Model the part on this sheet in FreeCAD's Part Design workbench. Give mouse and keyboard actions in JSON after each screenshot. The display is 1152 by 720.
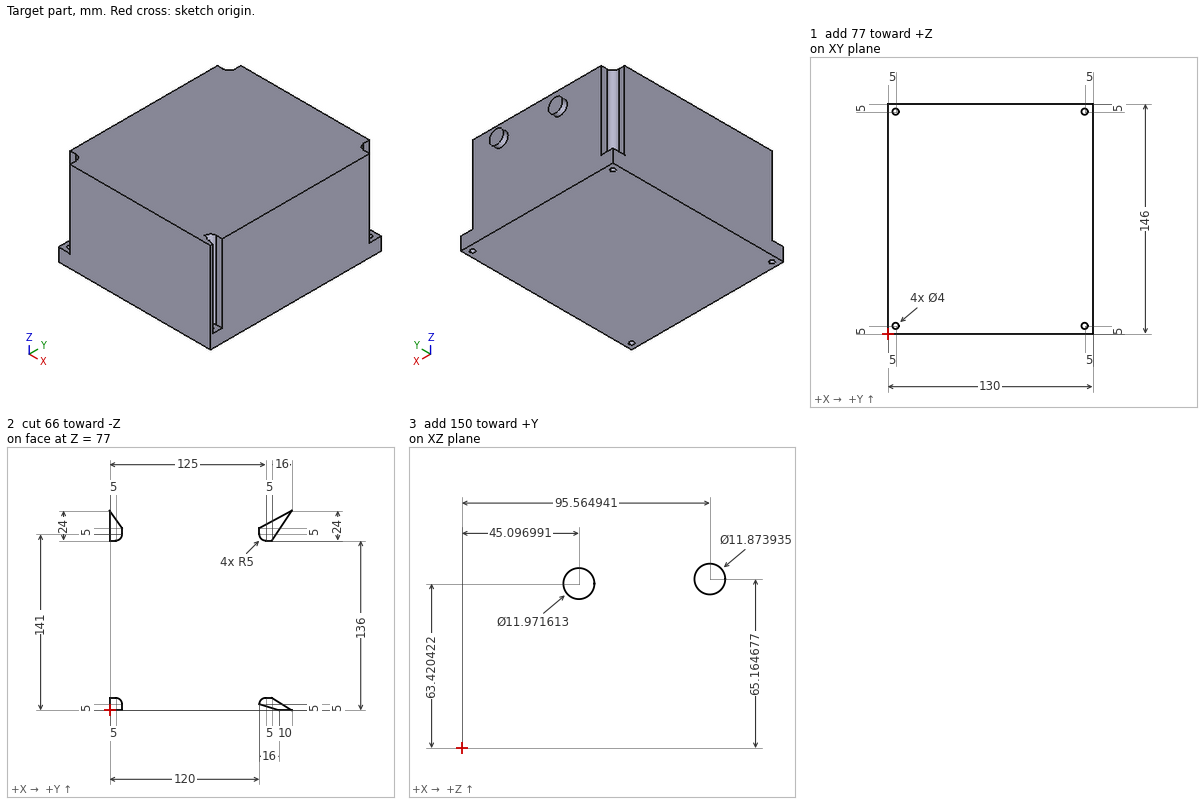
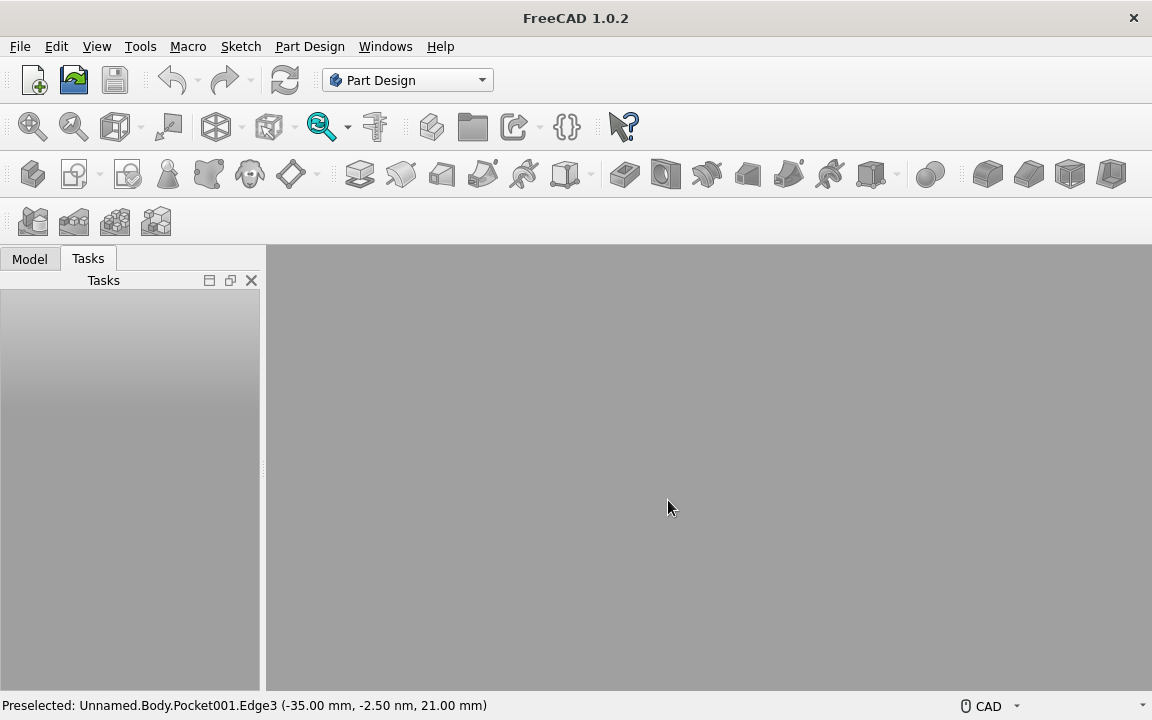
{"action": "left_click", "coordinate": [33, 80]}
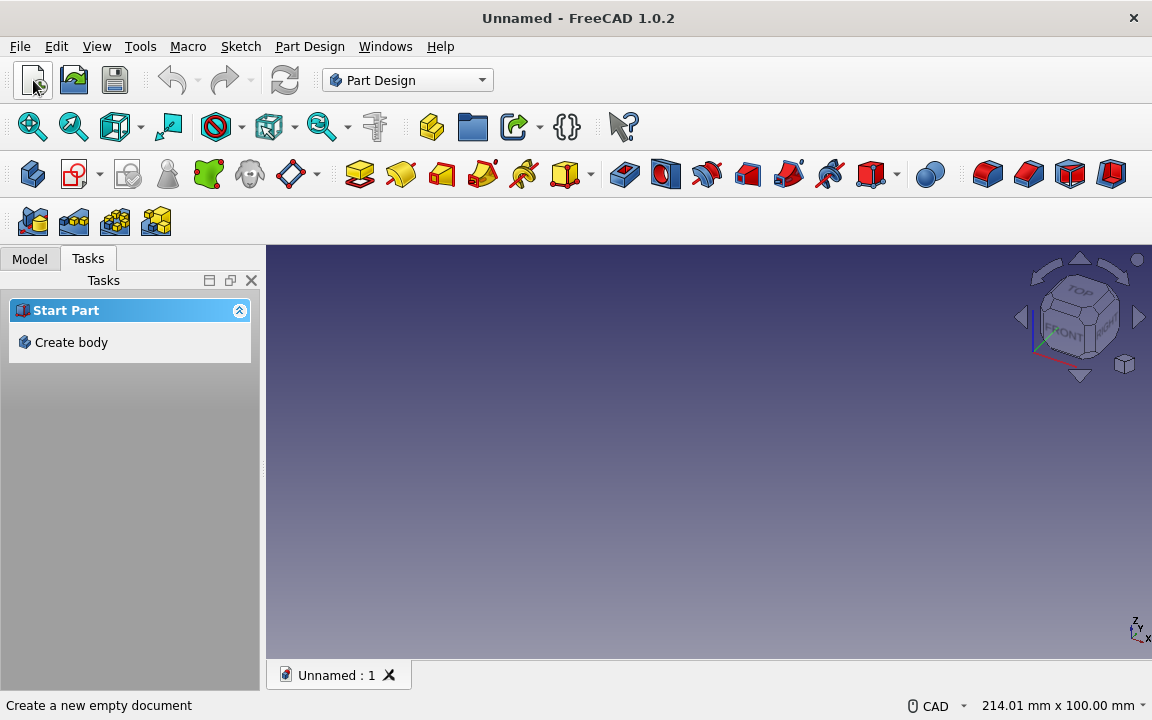
{"action": "left_click", "coordinate": [74, 174]}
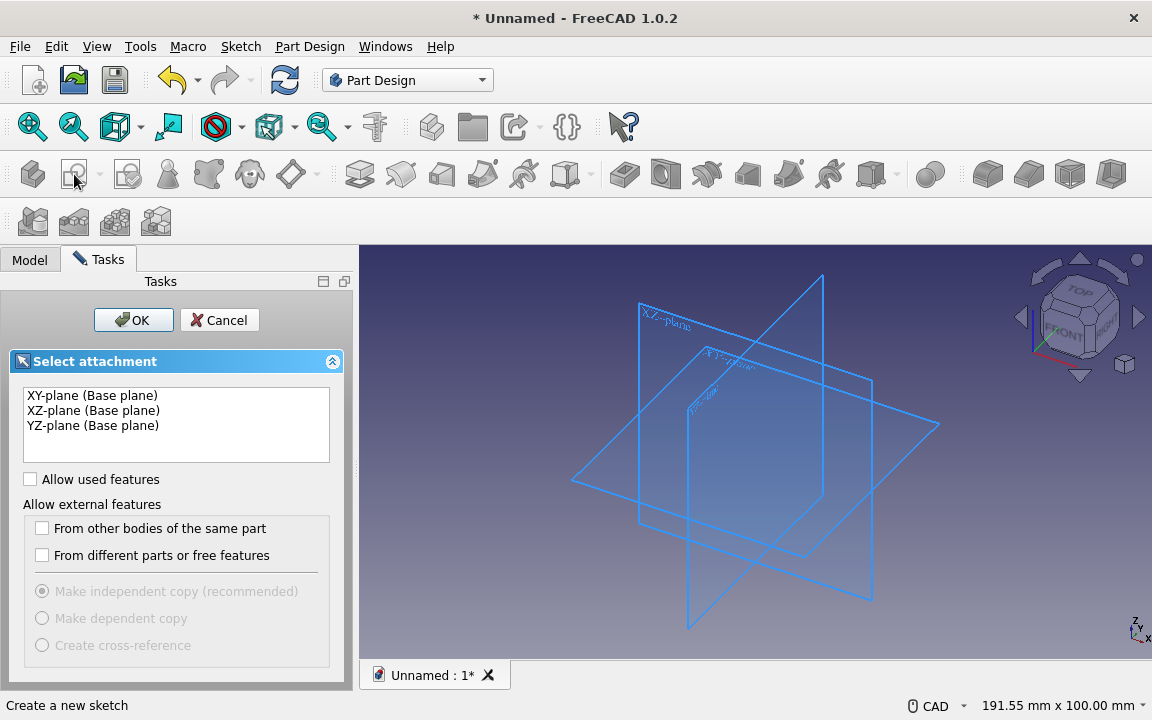
{"action": "left_click", "coordinate": [84, 396]}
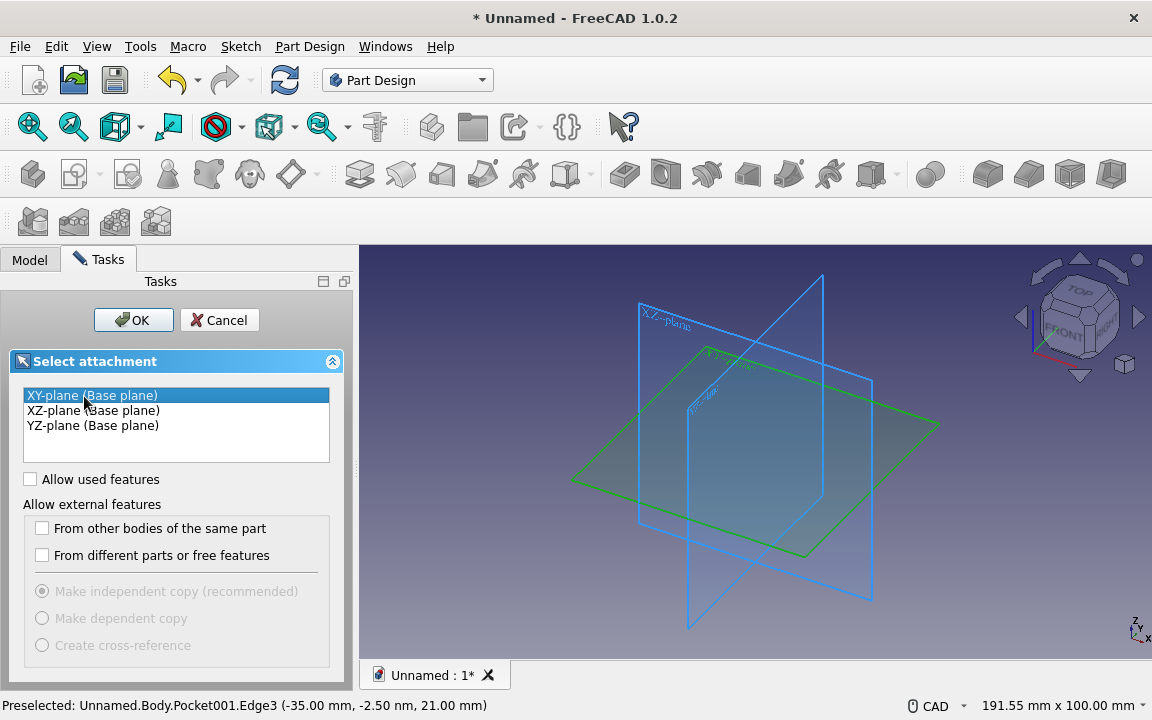
{"action": "left_click", "coordinate": [134, 320]}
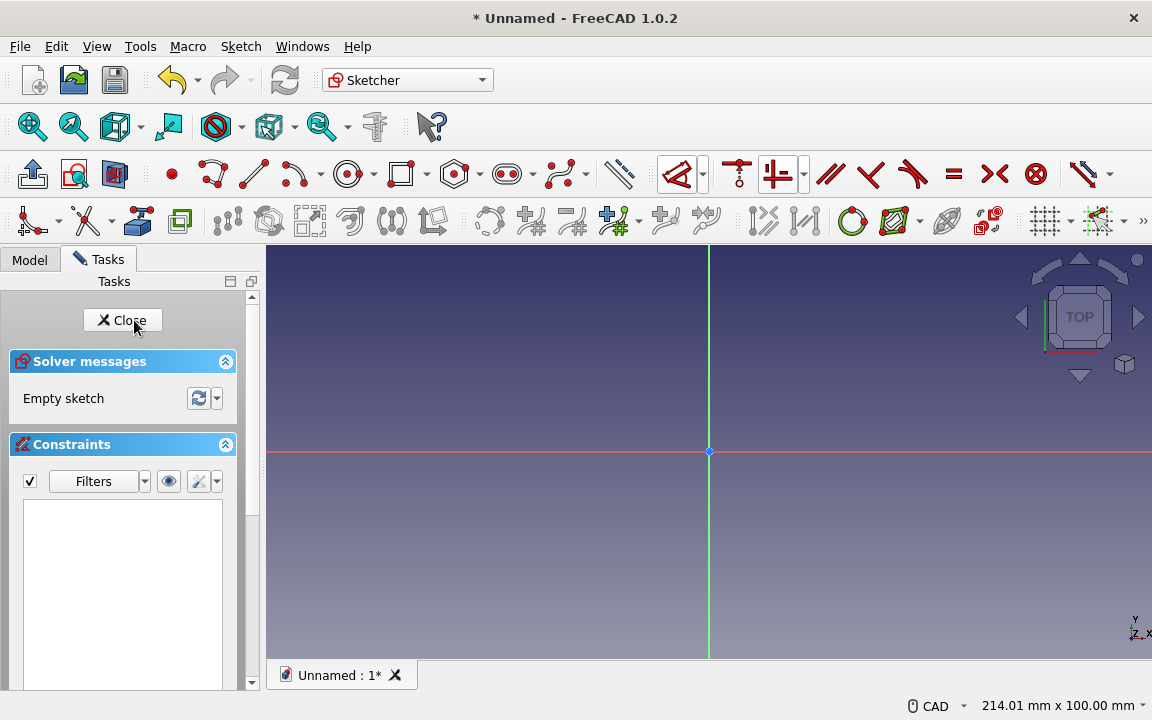
{"action": "scroll", "coordinate": [444, 628], "scroll_direction": "down", "scroll_amount": 5}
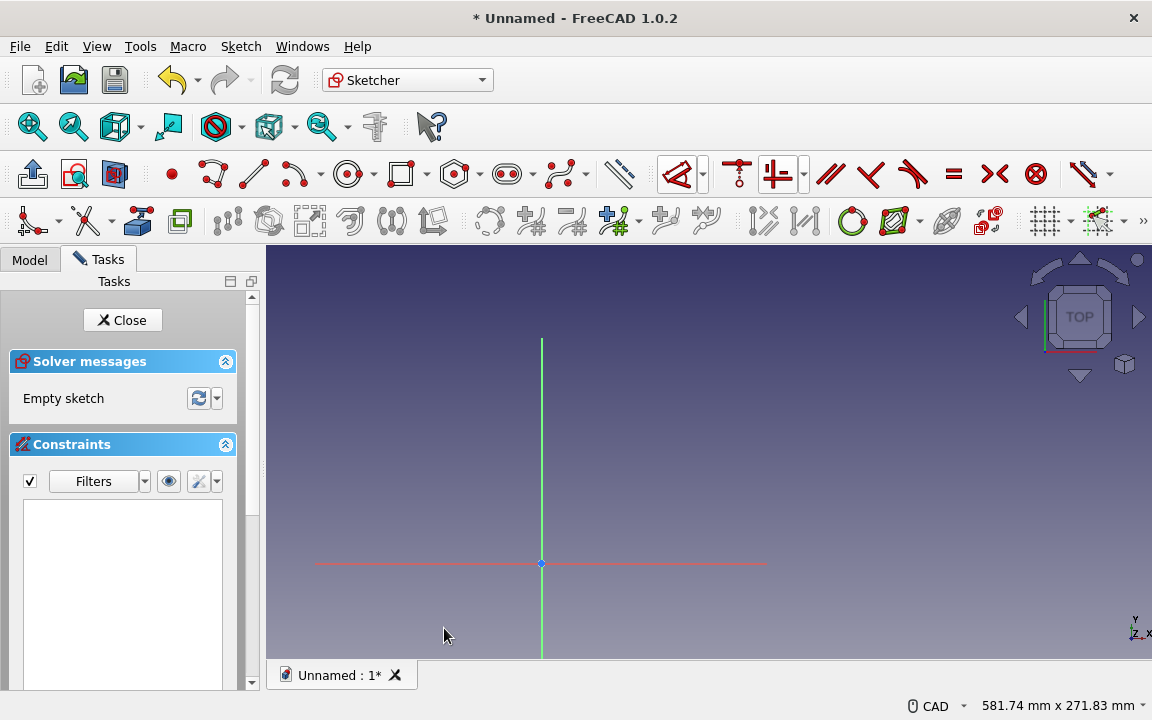
{"action": "left_click", "coordinate": [400, 174]}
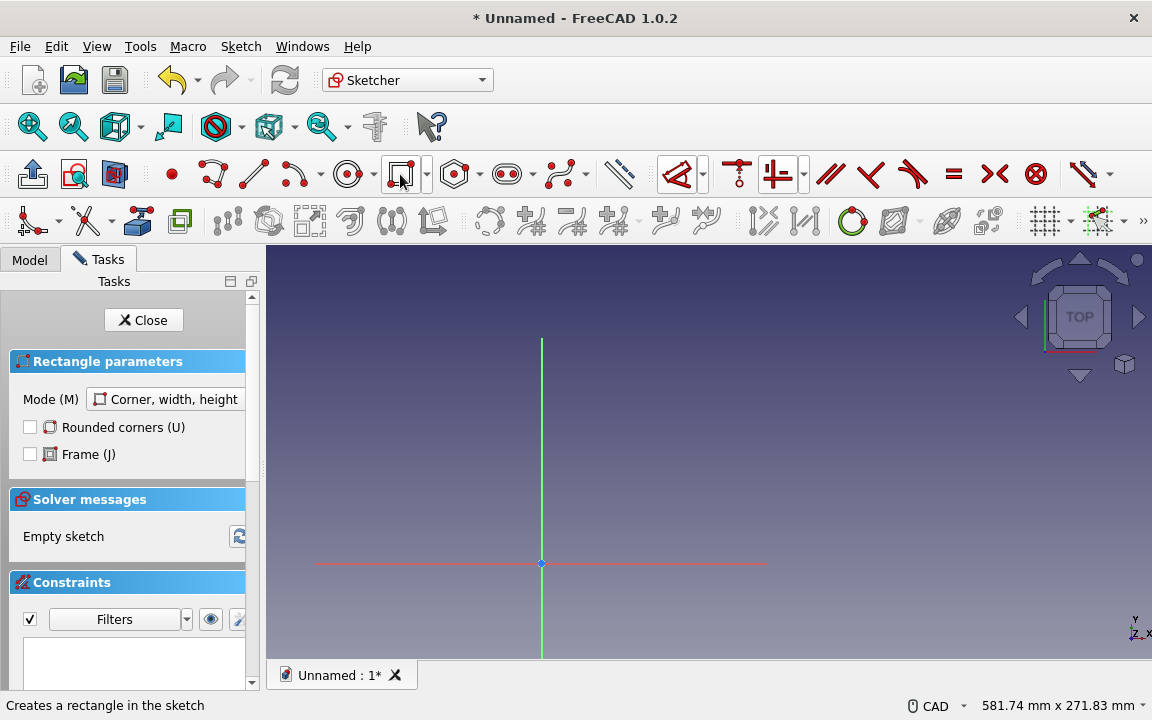
{"action": "left_click", "coordinate": [542, 564]}
{"action": "mouse_move", "coordinate": [740, 341]}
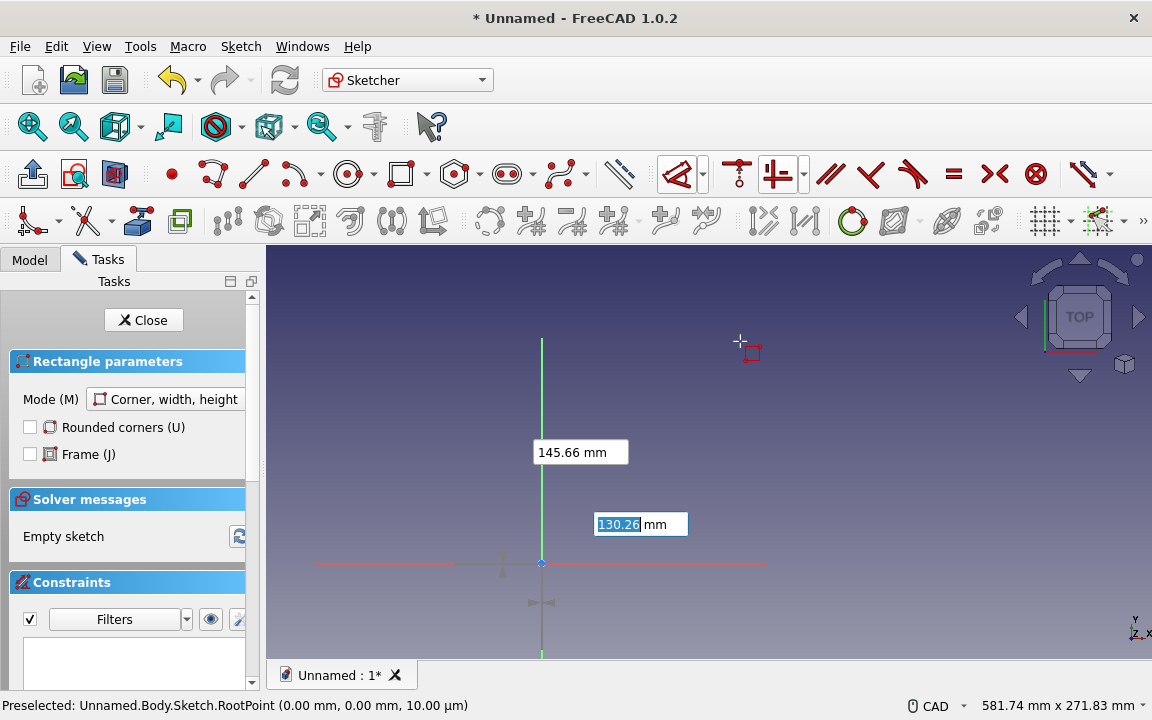
{"action": "type", "text": "130"}
{"action": "key", "text": "Tab"}
{"action": "type", "text": "146"}
{"action": "key", "text": "Return"}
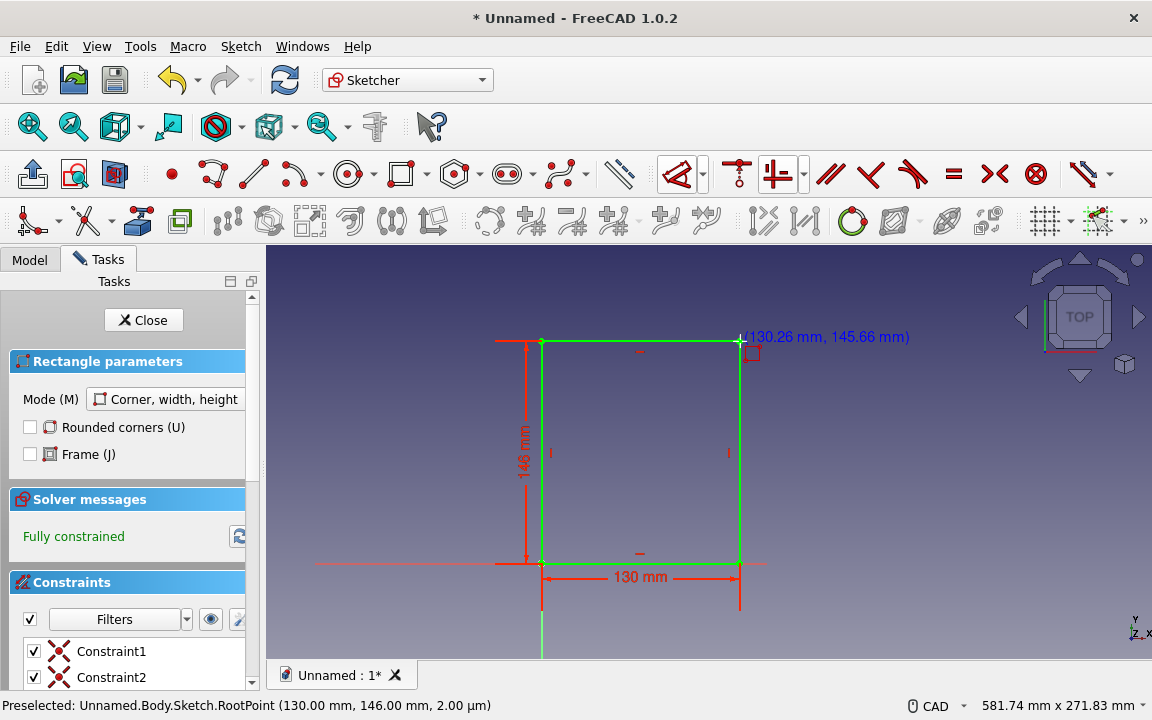
{"action": "left_click", "coordinate": [348, 174]}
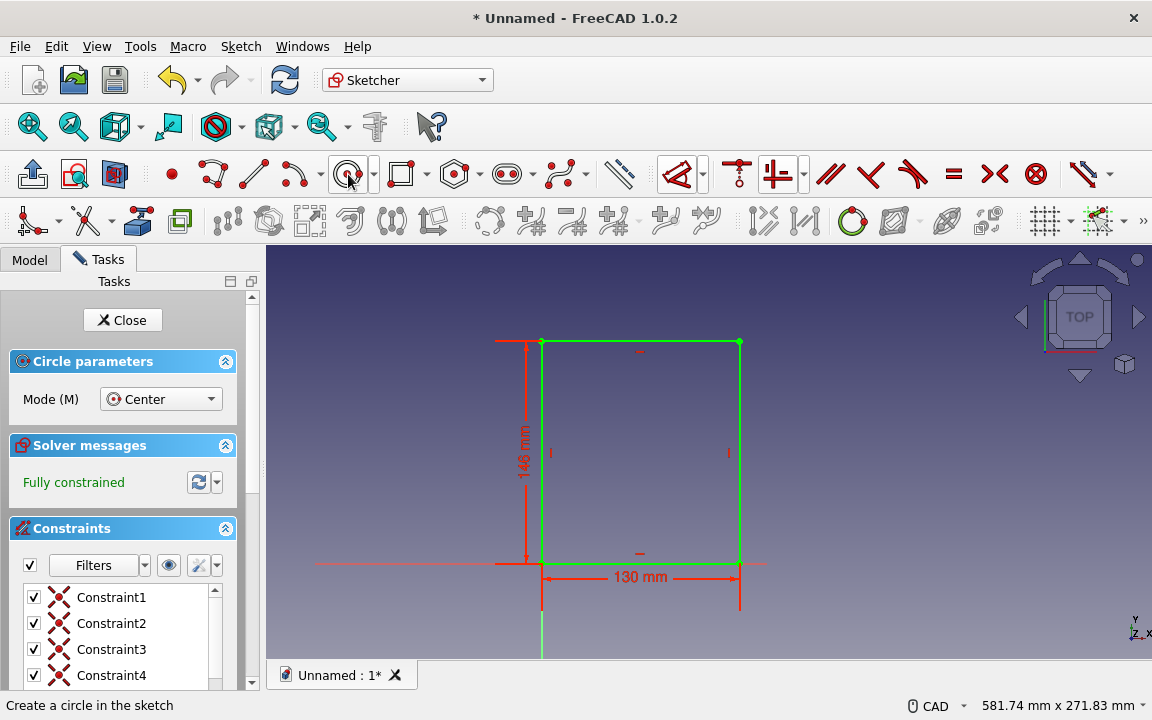
{"action": "scroll", "coordinate": [549, 556], "scroll_direction": "up", "scroll_amount": 11}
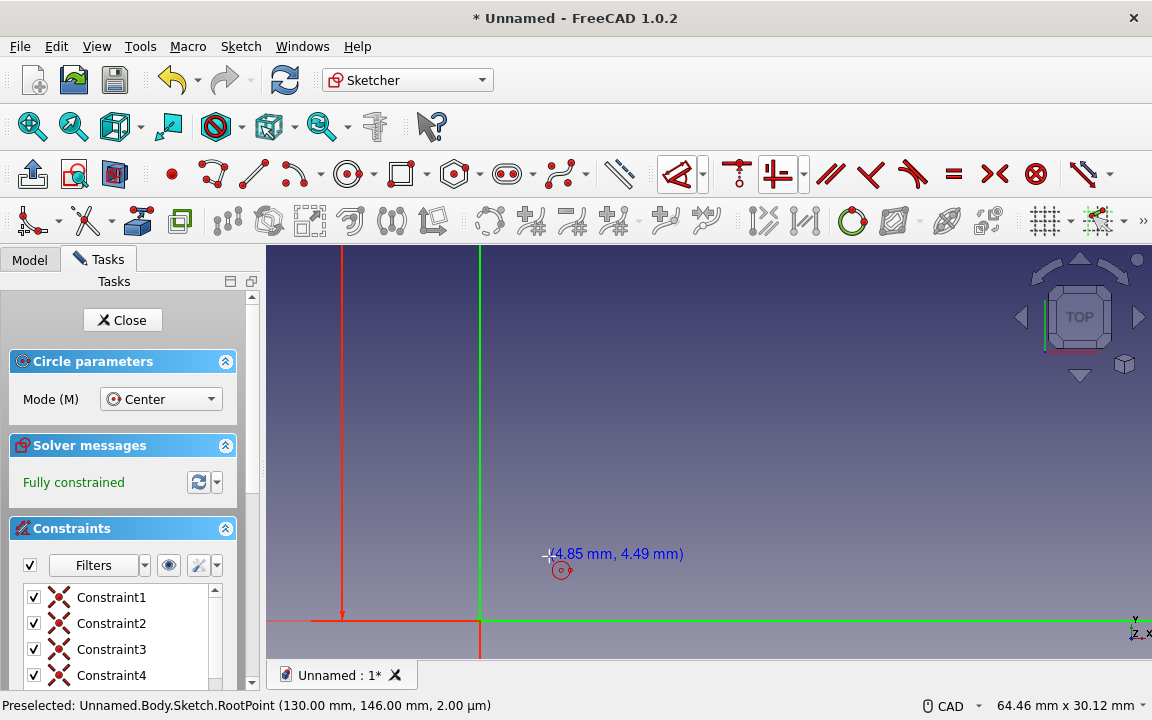
{"action": "scroll", "coordinate": [526, 583], "scroll_direction": "down", "scroll_amount": 10}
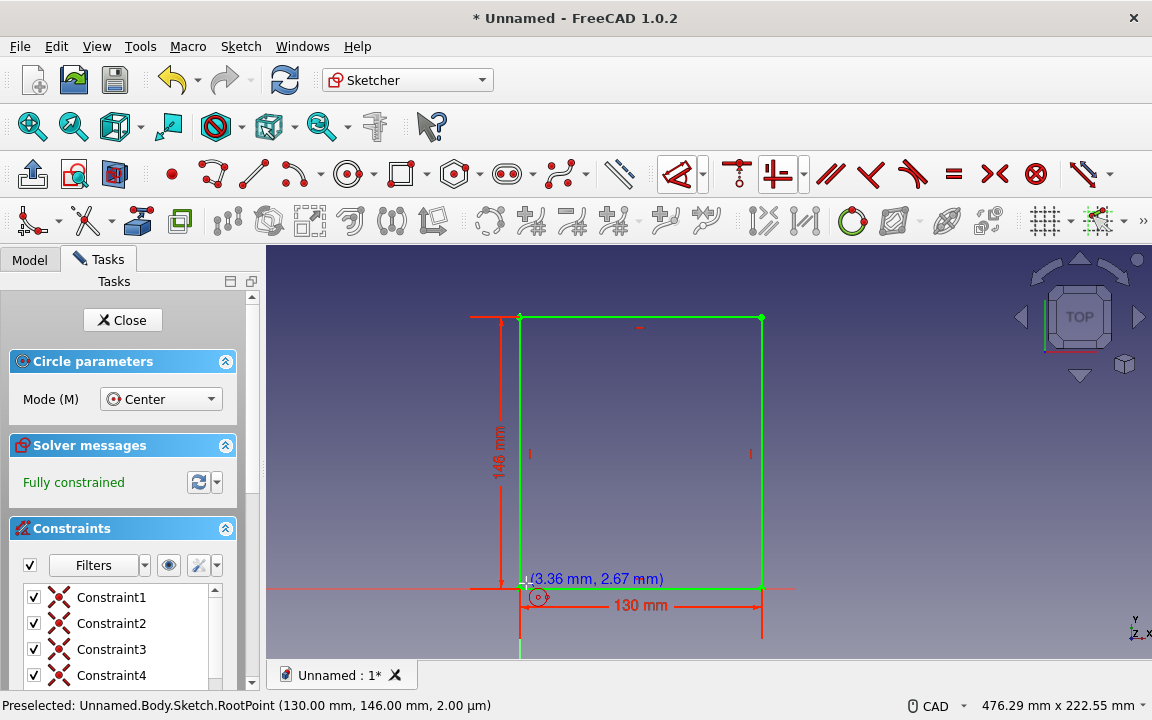
{"action": "scroll", "coordinate": [529, 580], "scroll_direction": "up", "scroll_amount": 3}